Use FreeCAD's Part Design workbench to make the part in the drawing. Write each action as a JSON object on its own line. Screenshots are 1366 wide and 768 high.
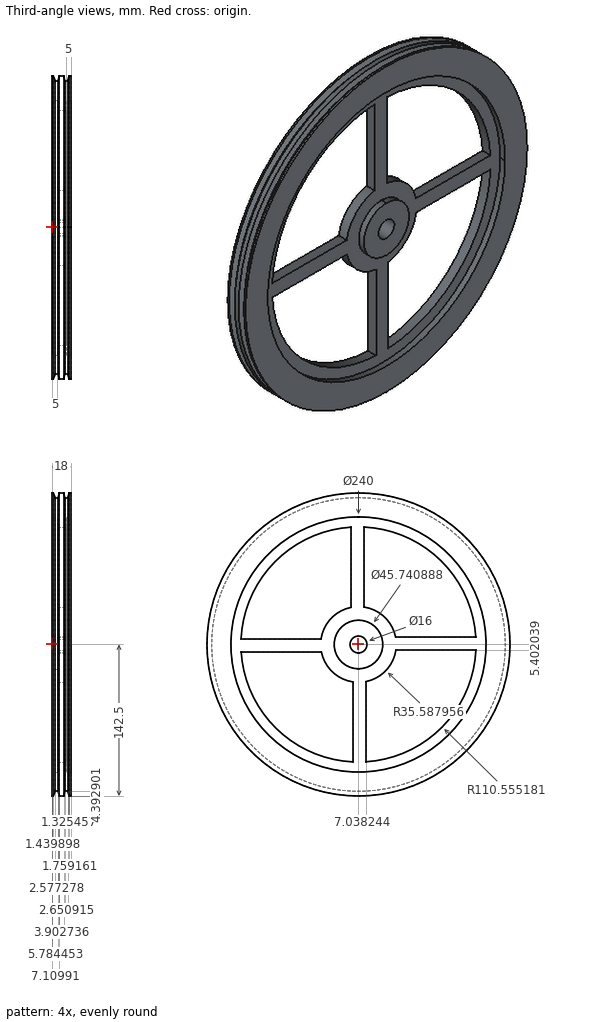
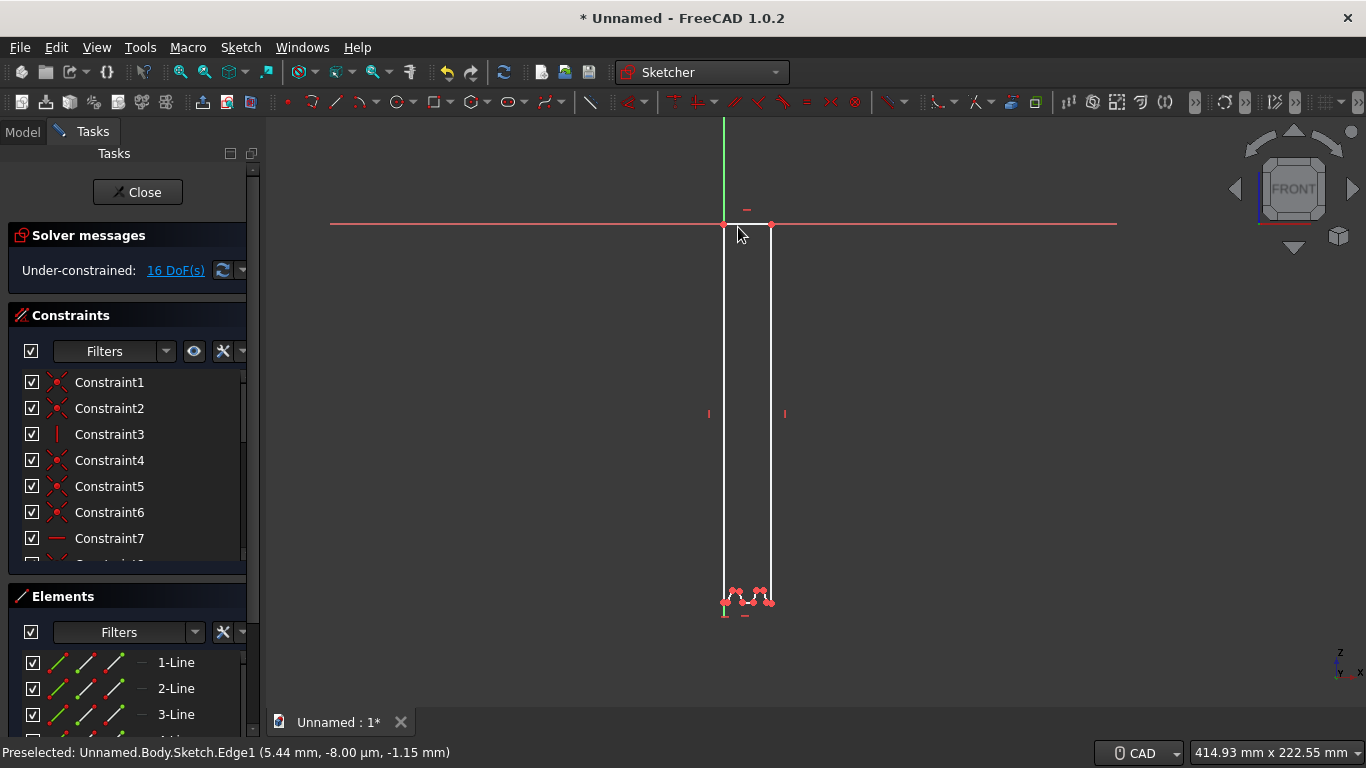
{"action": "scroll", "coordinate": [769, 603], "scroll_direction": "up", "scroll_amount": 10}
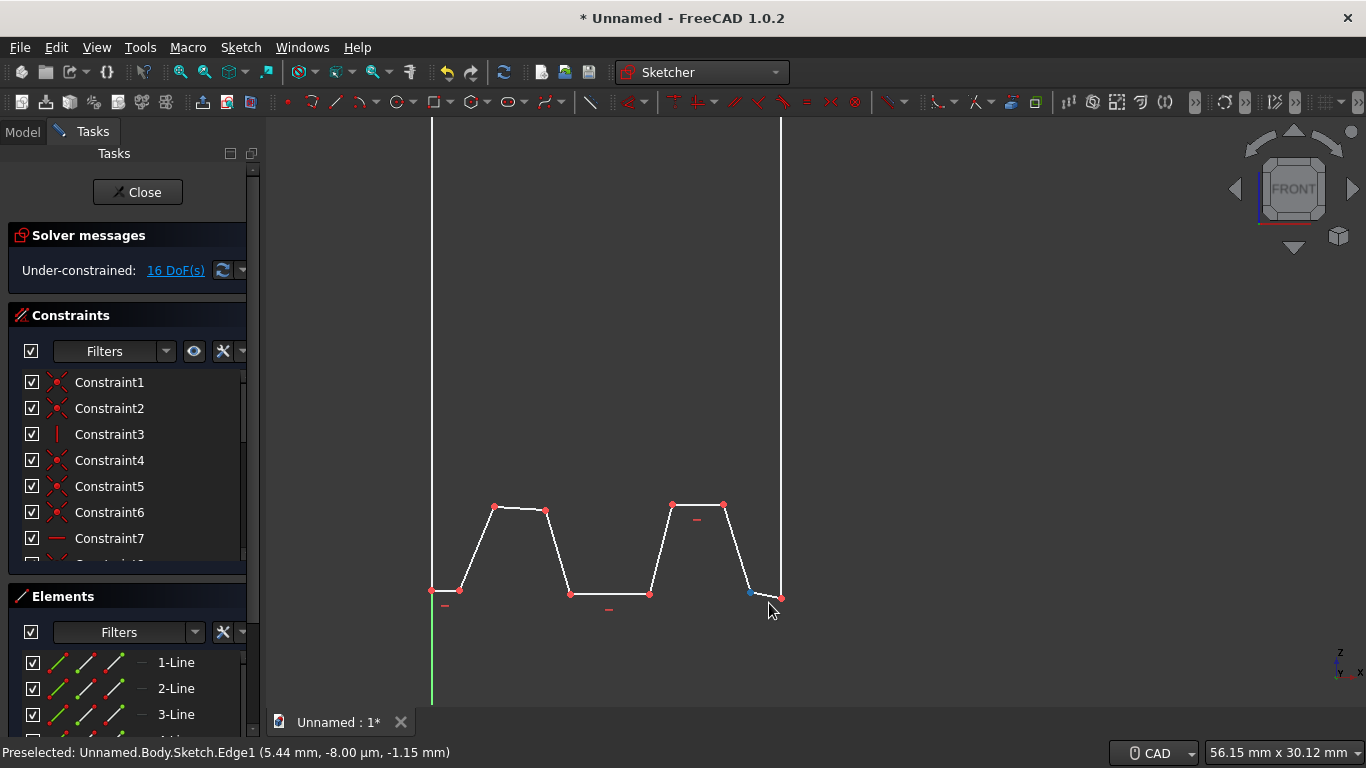
{"action": "left_click", "coordinate": [766, 595]}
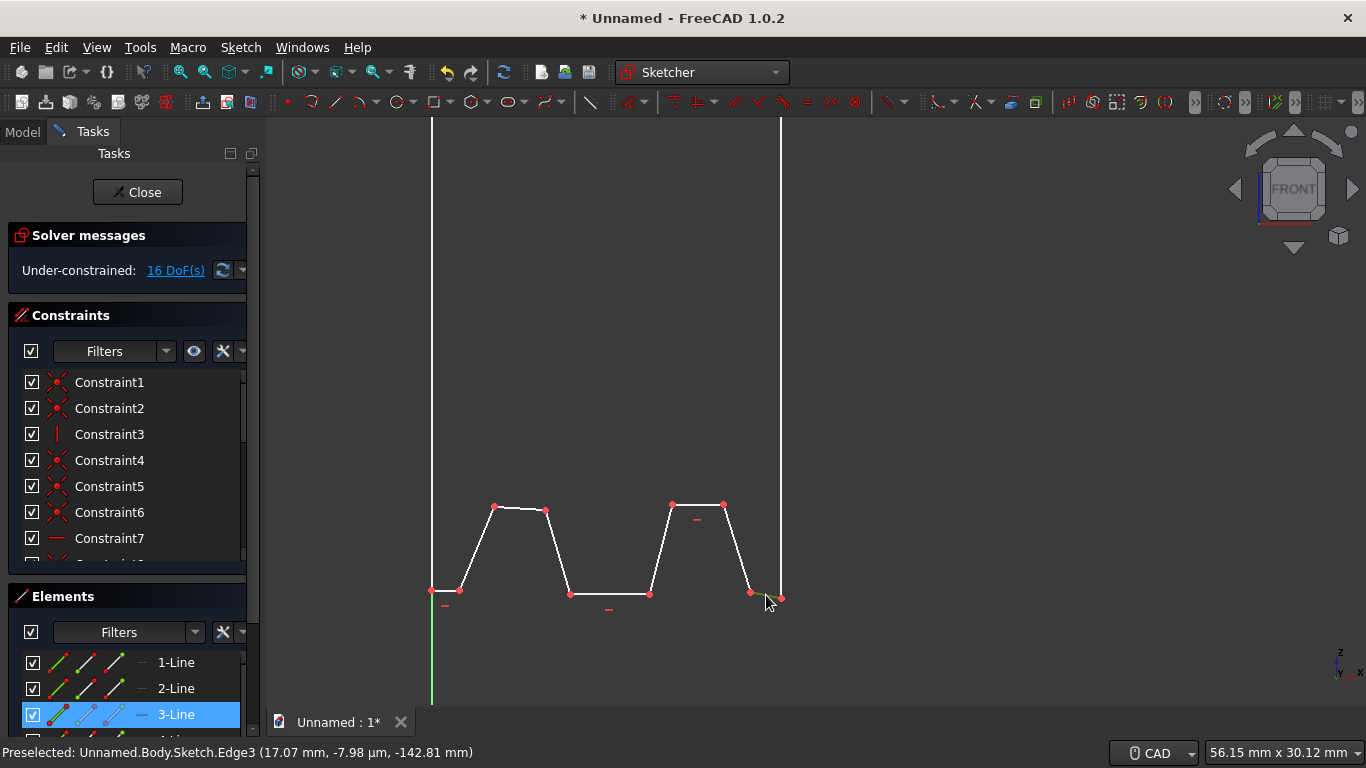
{"action": "key", "text": "h"}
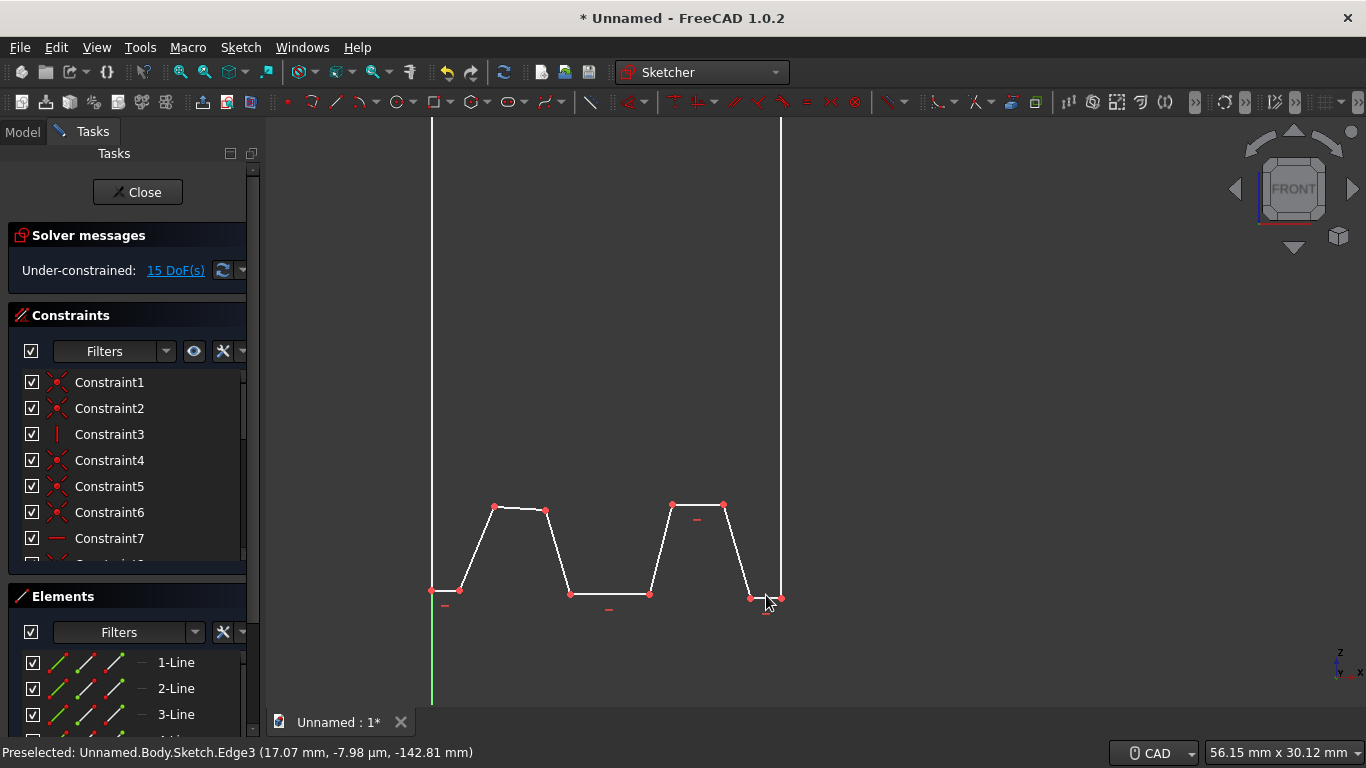
{"action": "left_click", "coordinate": [530, 509]}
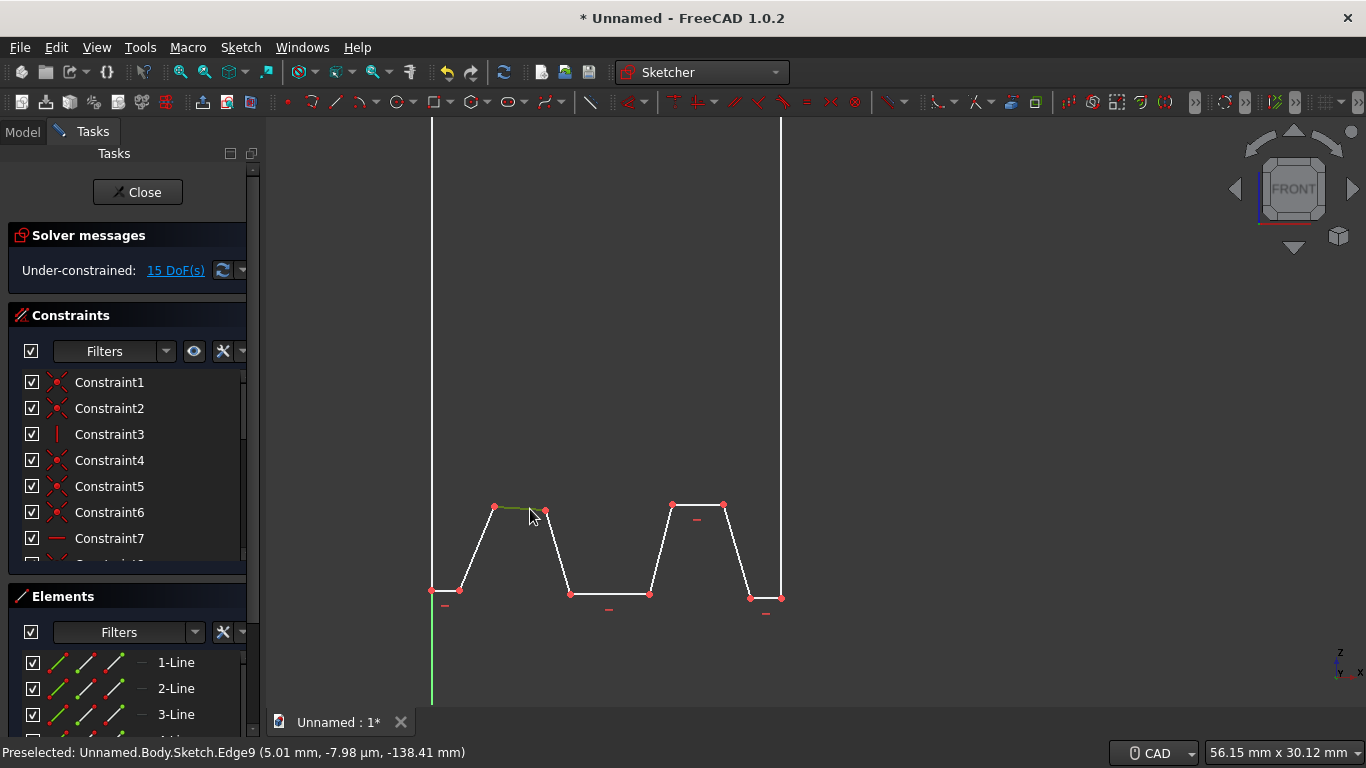
{"action": "key", "text": "h"}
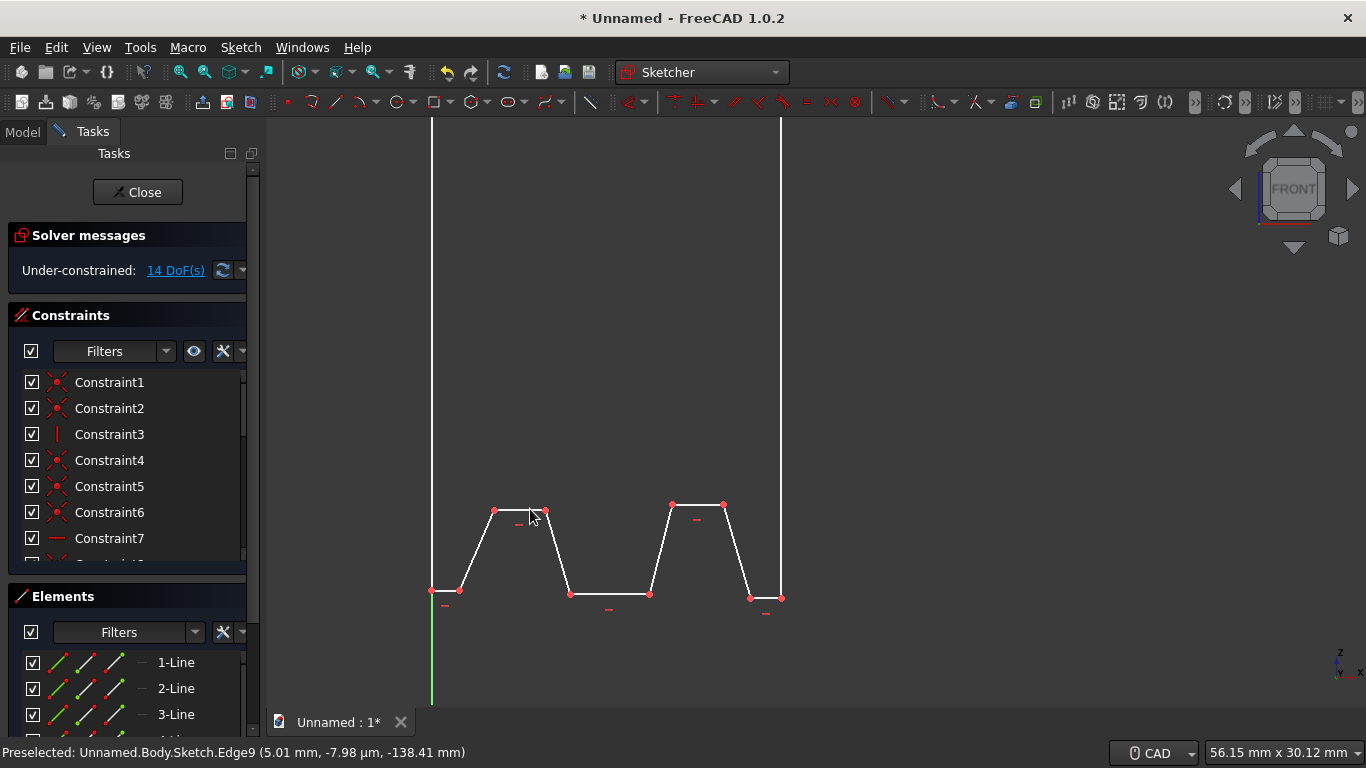
{"action": "key", "text": "d"}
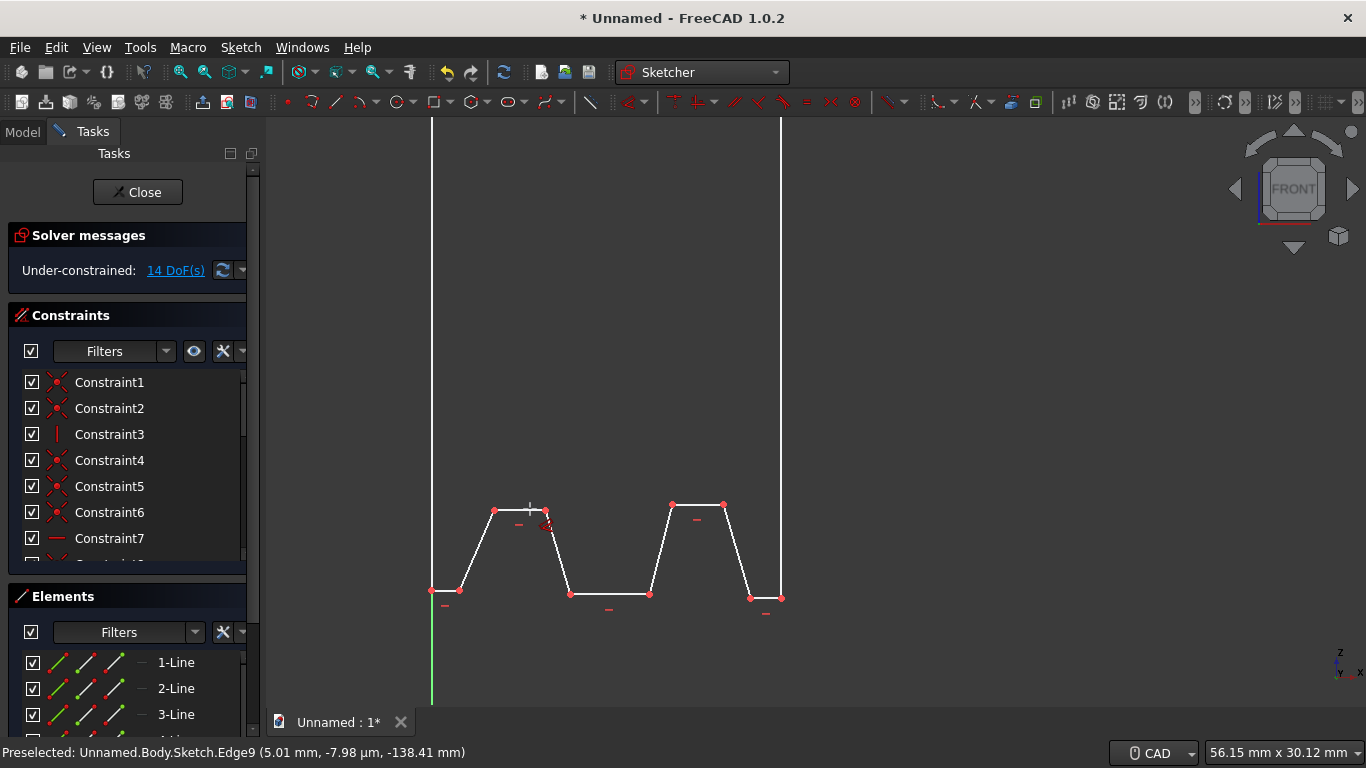
{"action": "scroll", "coordinate": [769, 603], "scroll_direction": "down", "scroll_amount": 10}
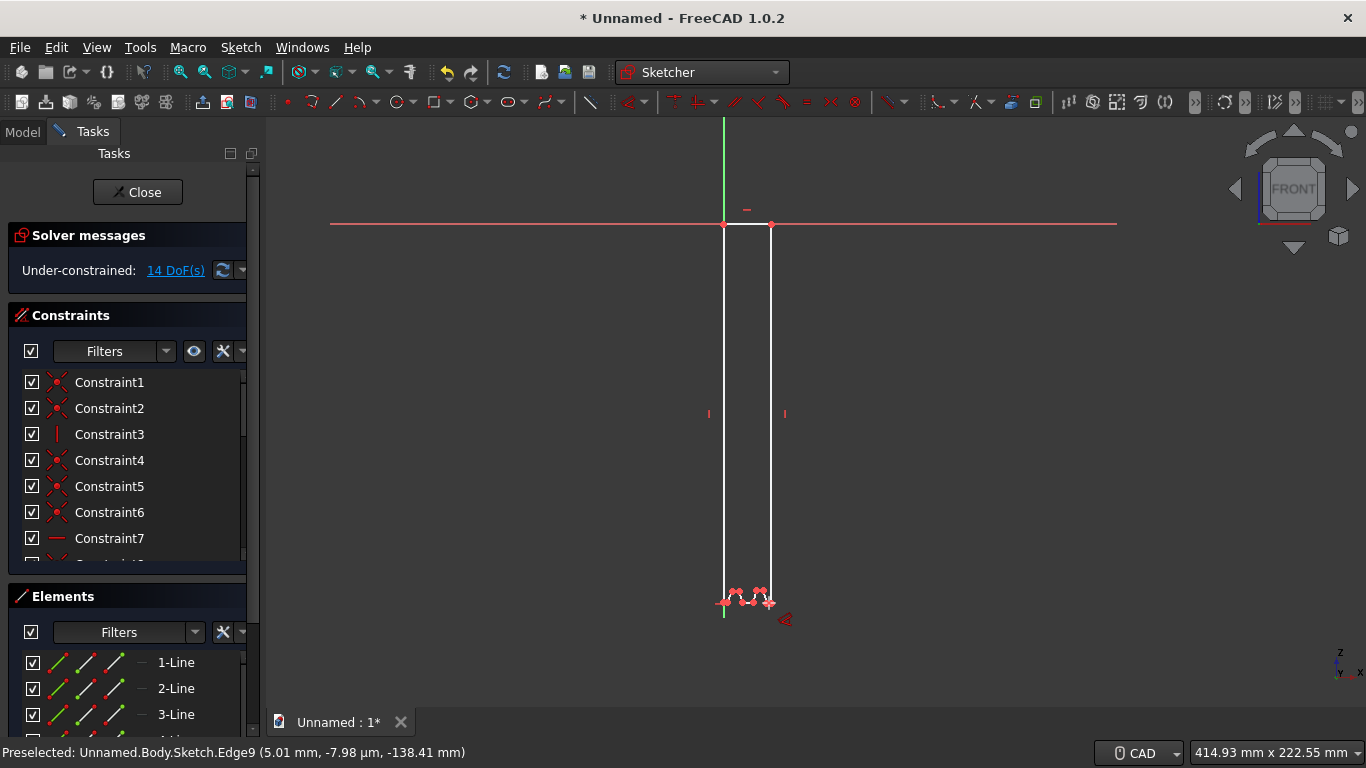
{"action": "left_click", "coordinate": [738, 224]}
{"action": "left_click", "coordinate": [747, 190]}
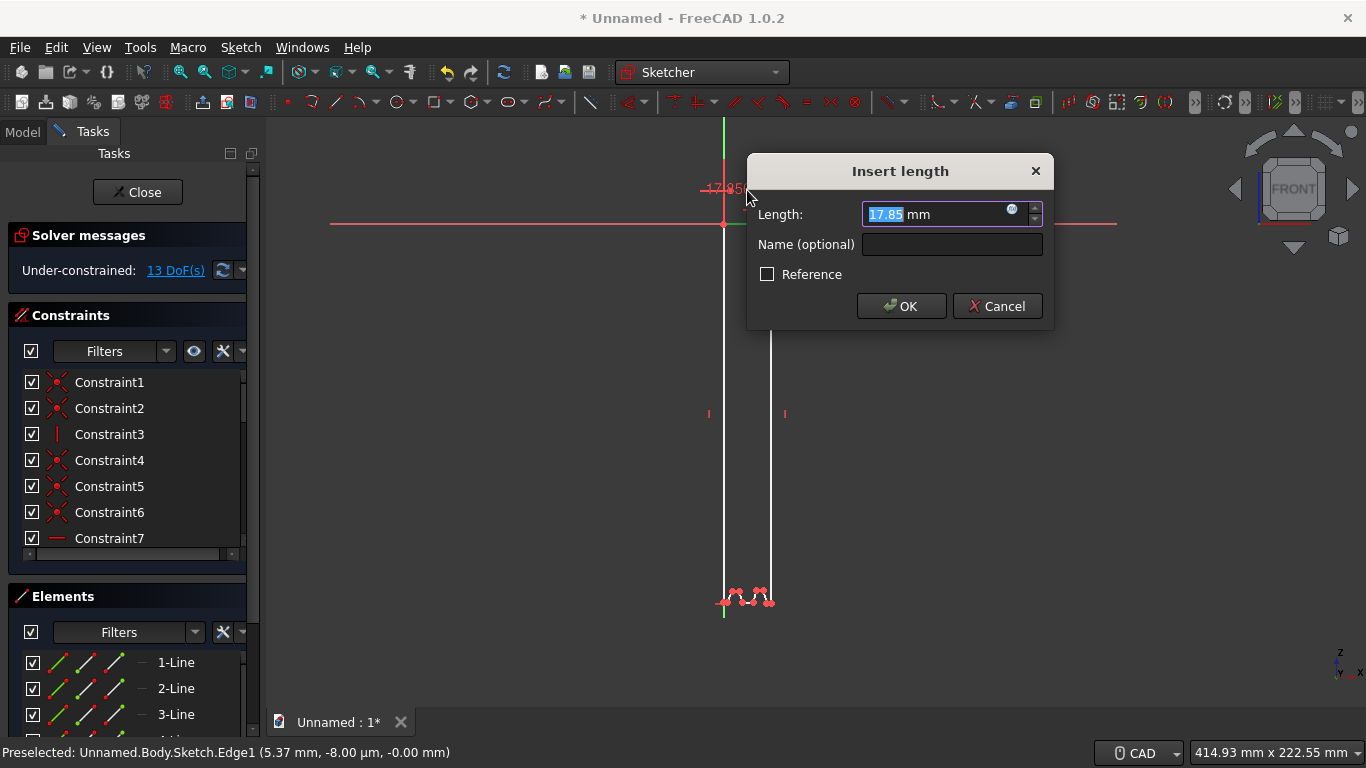
{"action": "type", "text": "18"}
{"action": "key", "text": "Return"}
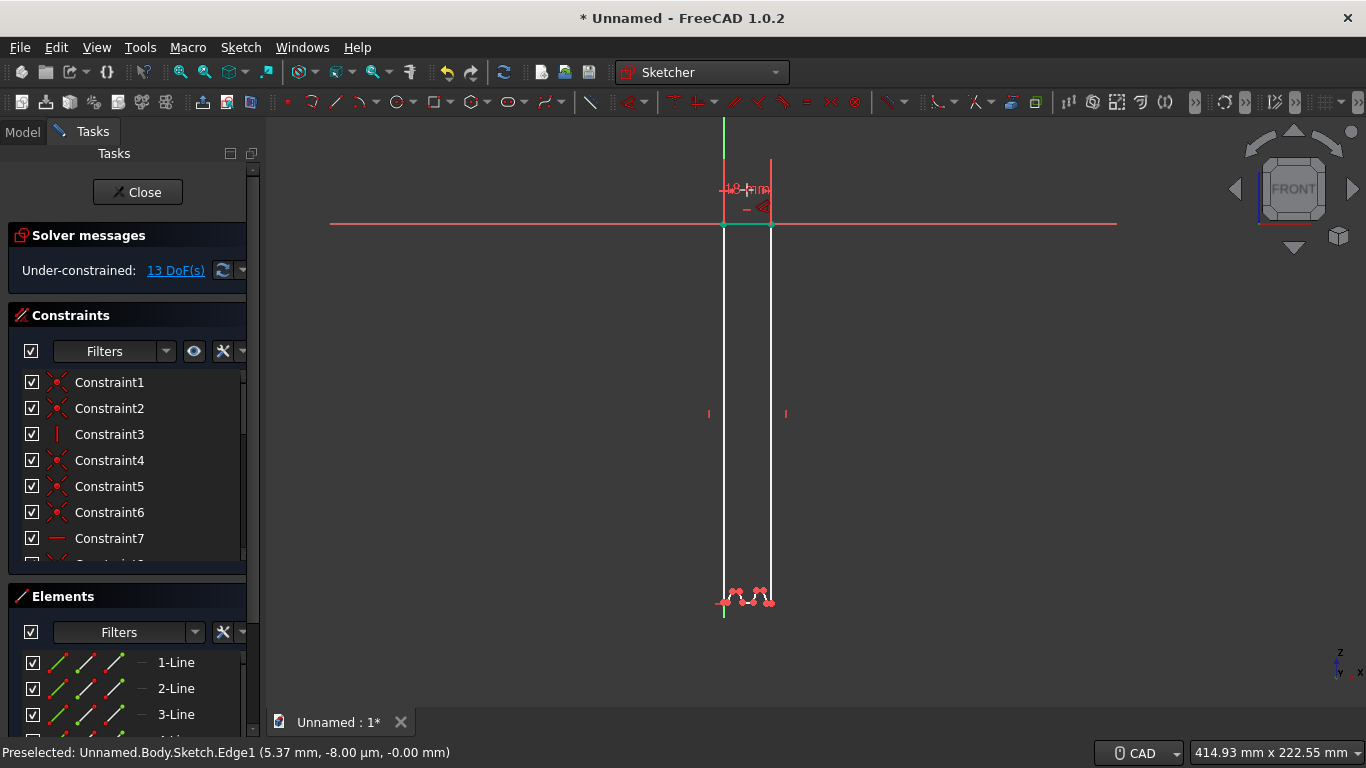
{"action": "left_click", "coordinate": [771, 338]}
{"action": "left_click", "coordinate": [805, 414]}